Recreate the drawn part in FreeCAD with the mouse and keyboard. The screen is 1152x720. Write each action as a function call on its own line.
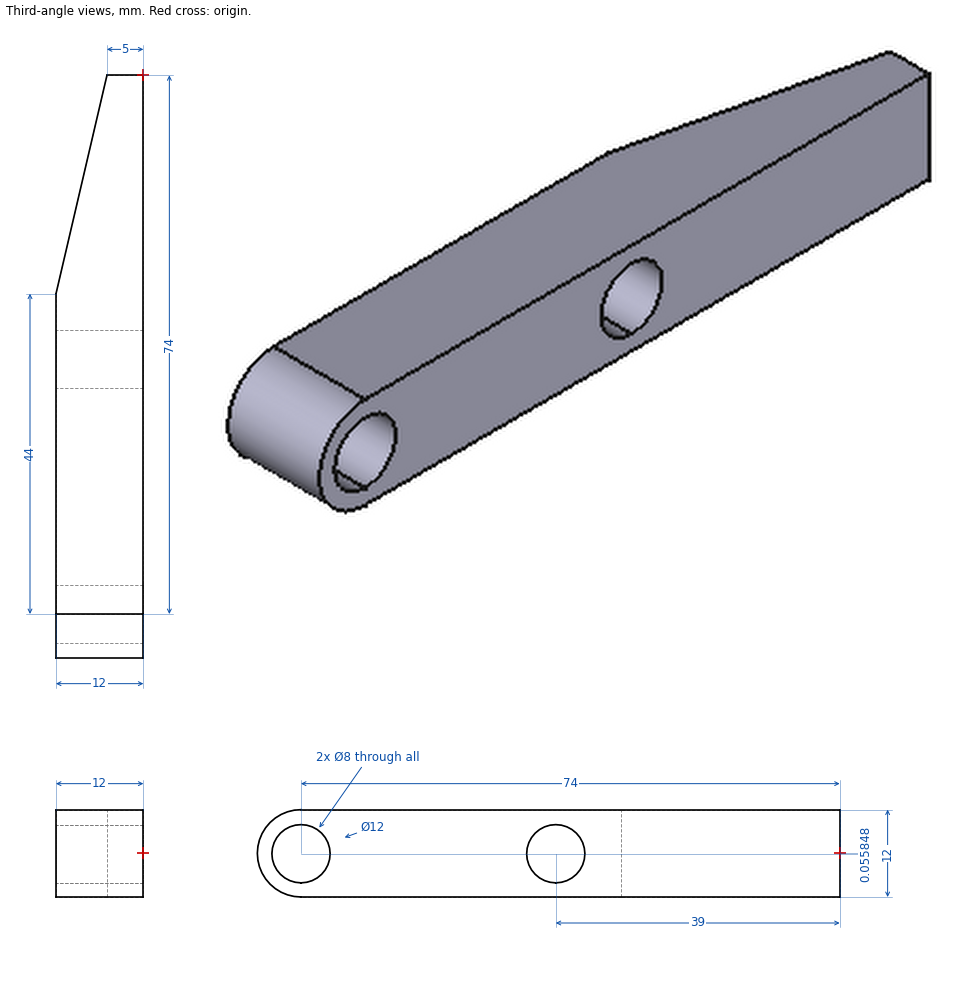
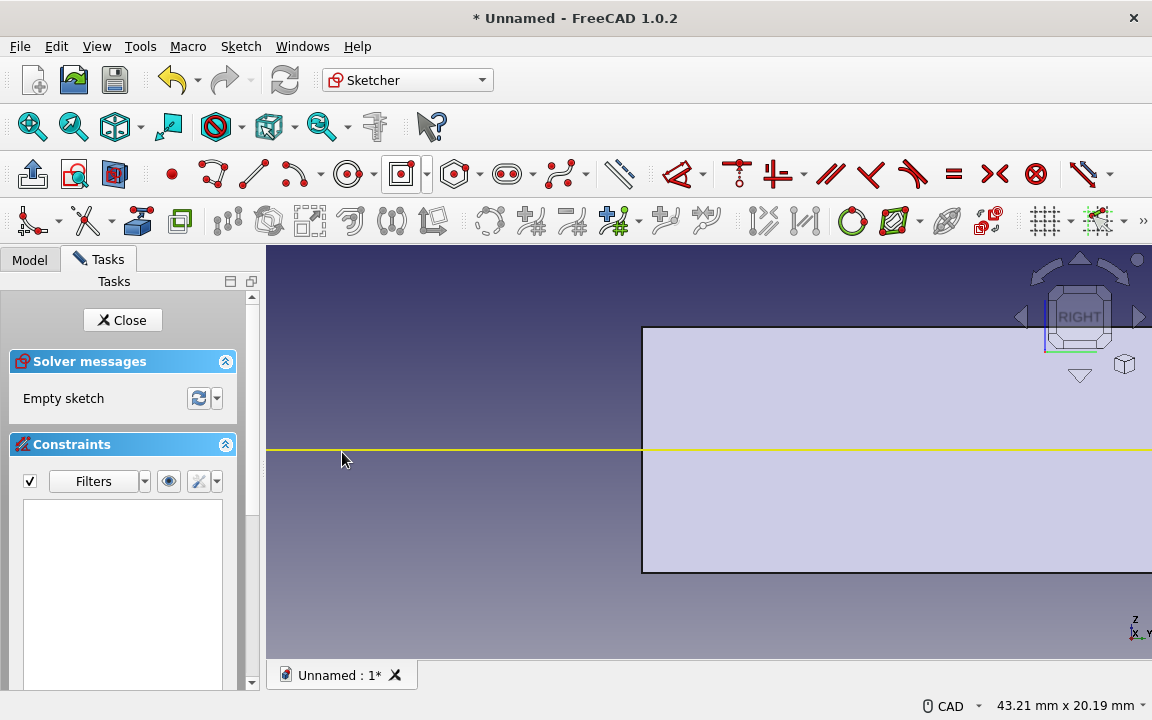
key(g)
key(c)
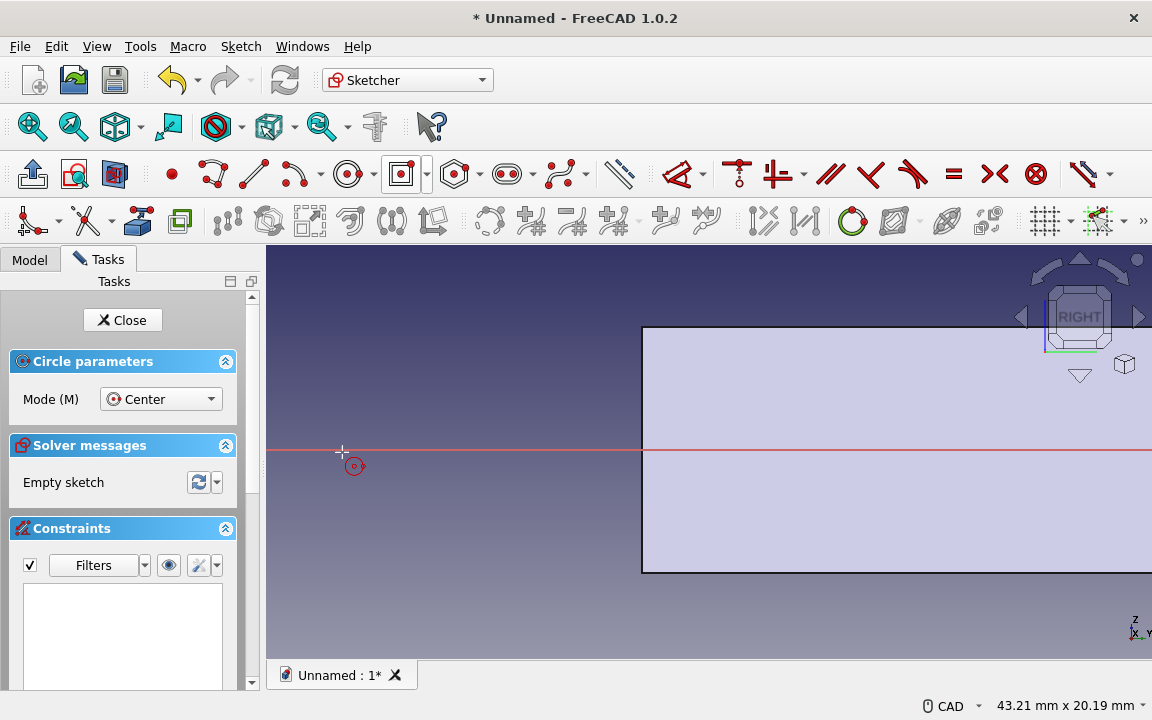
click(642, 450)
move(729, 363)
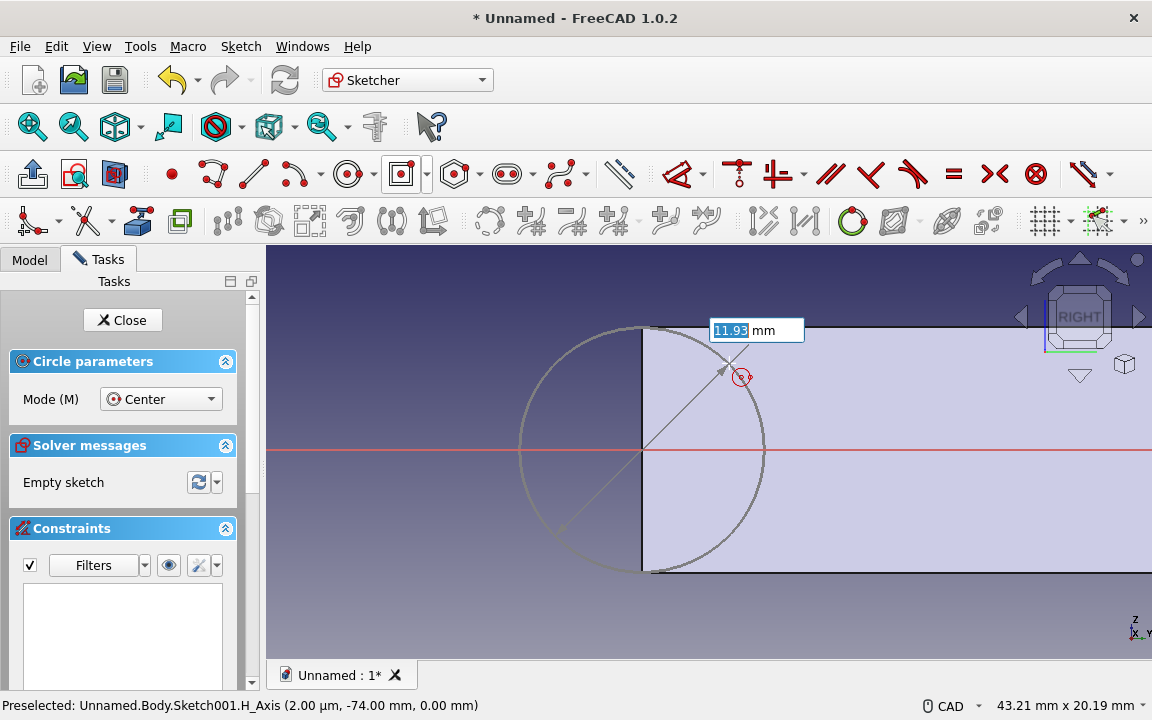
text(12)
key(Return)
key(Escape)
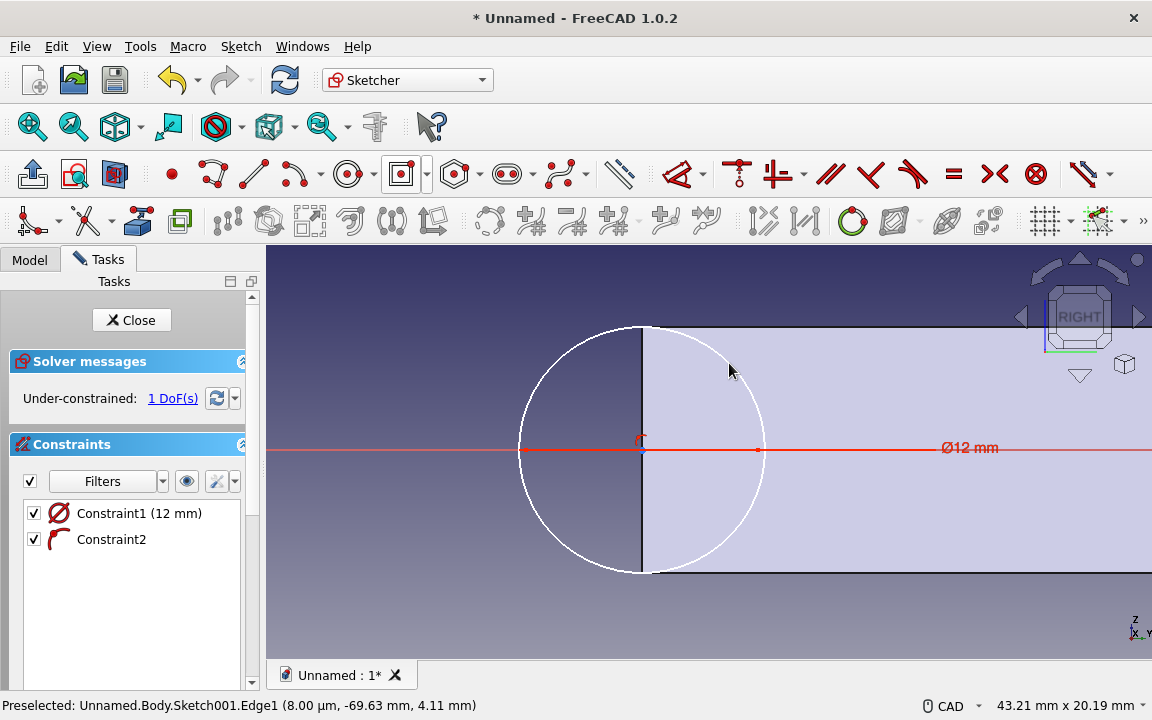
click(642, 450)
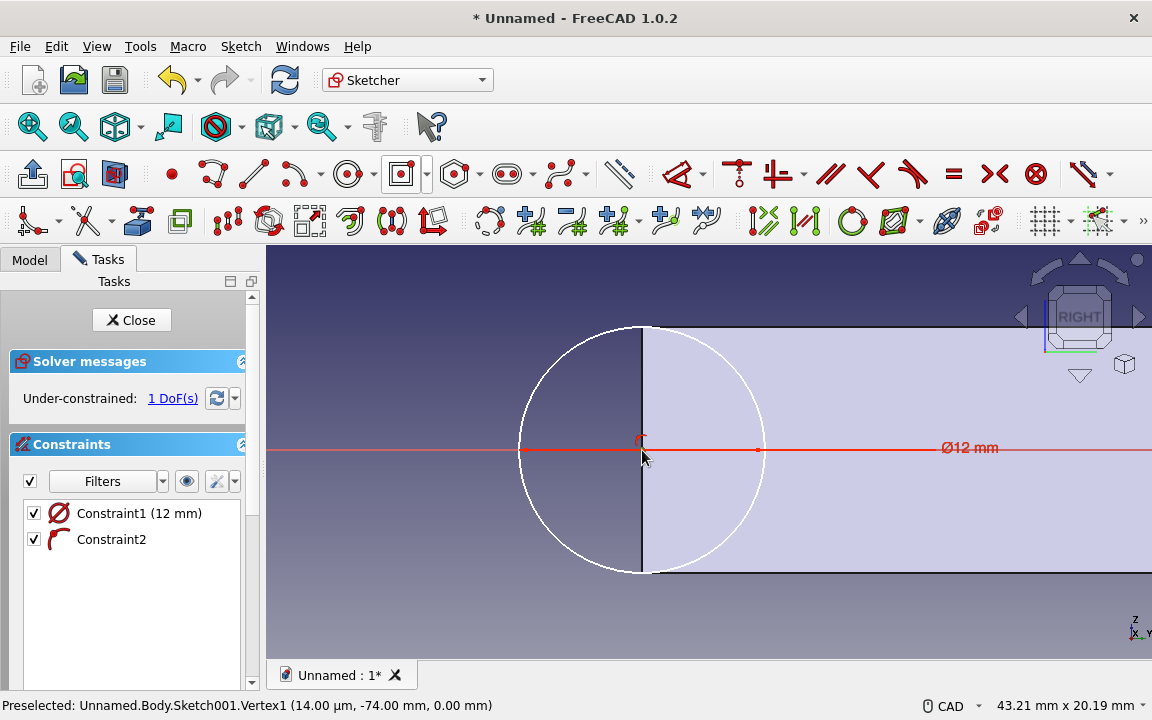
key(l)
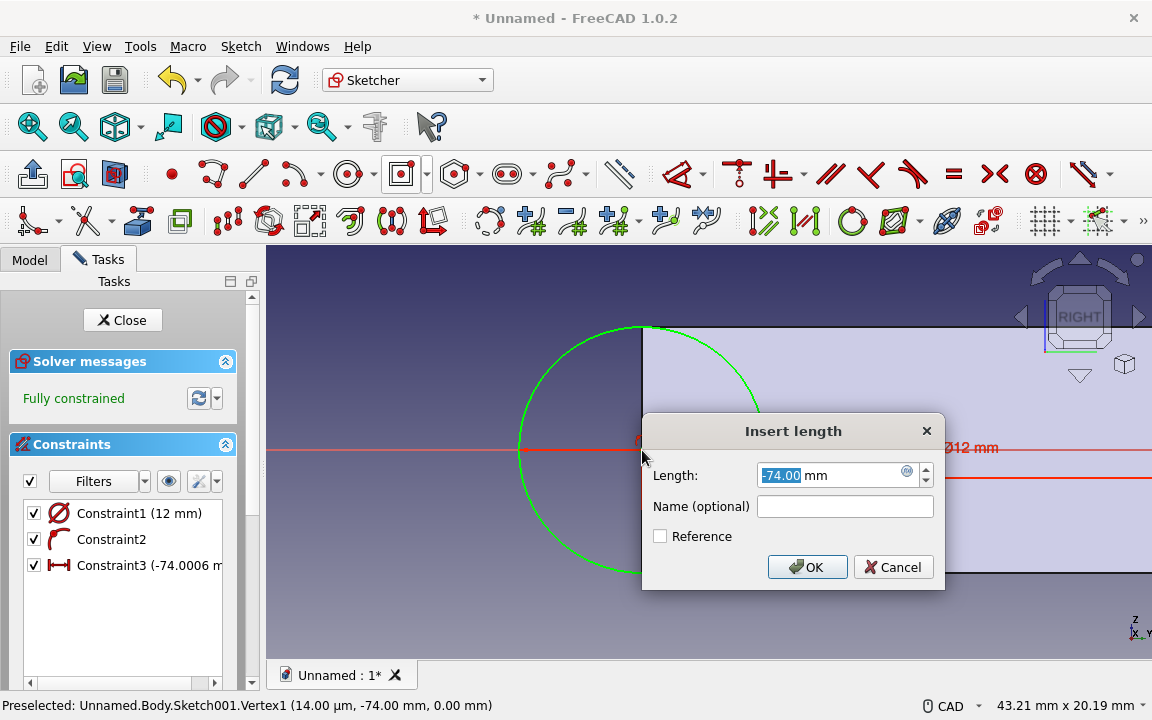
text(-74)
key(Return)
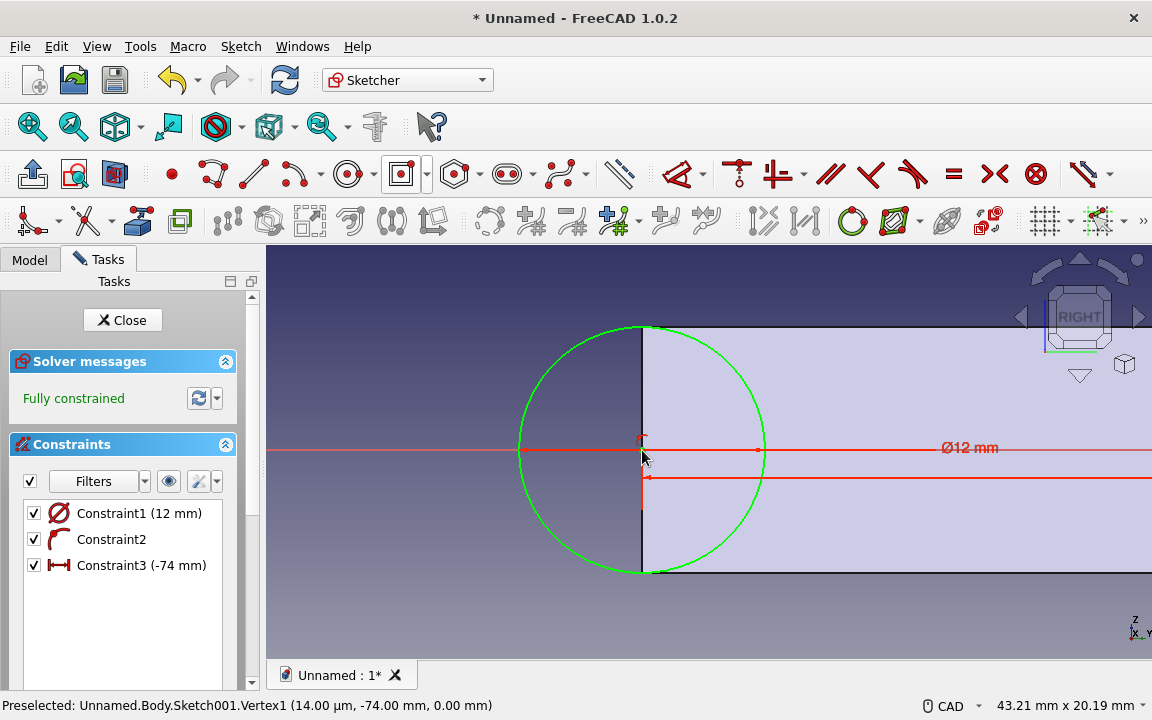
click(123, 320)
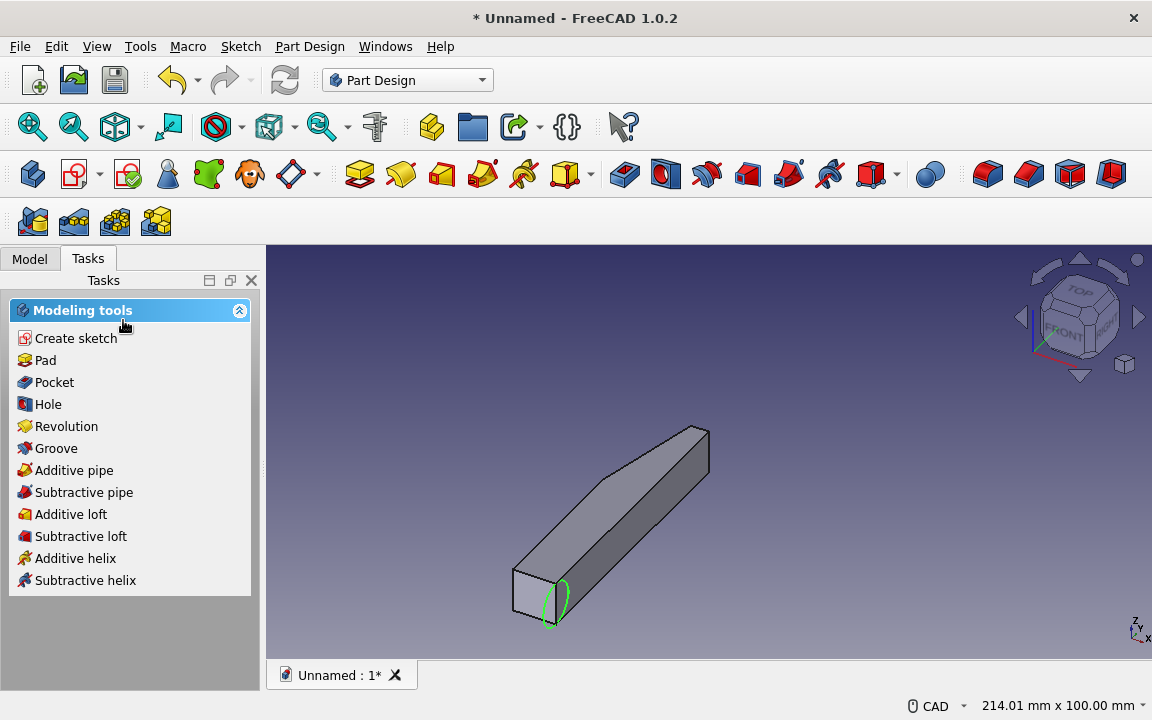
click(360, 174)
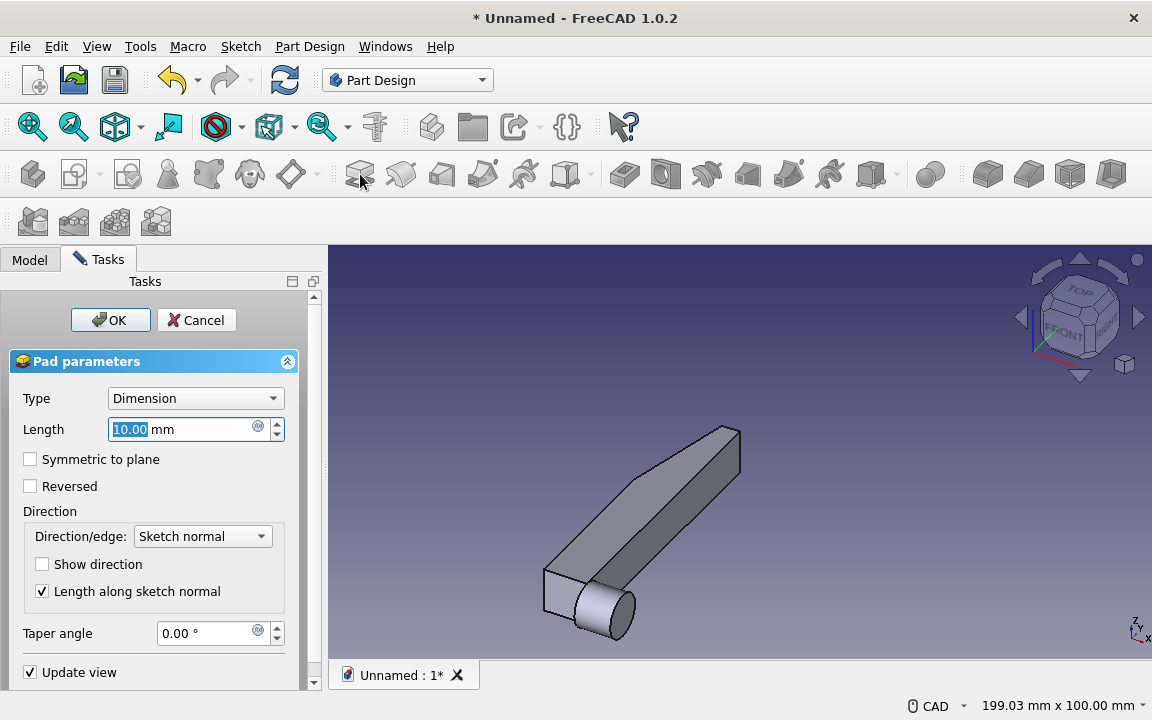
text(12)
key(Tab)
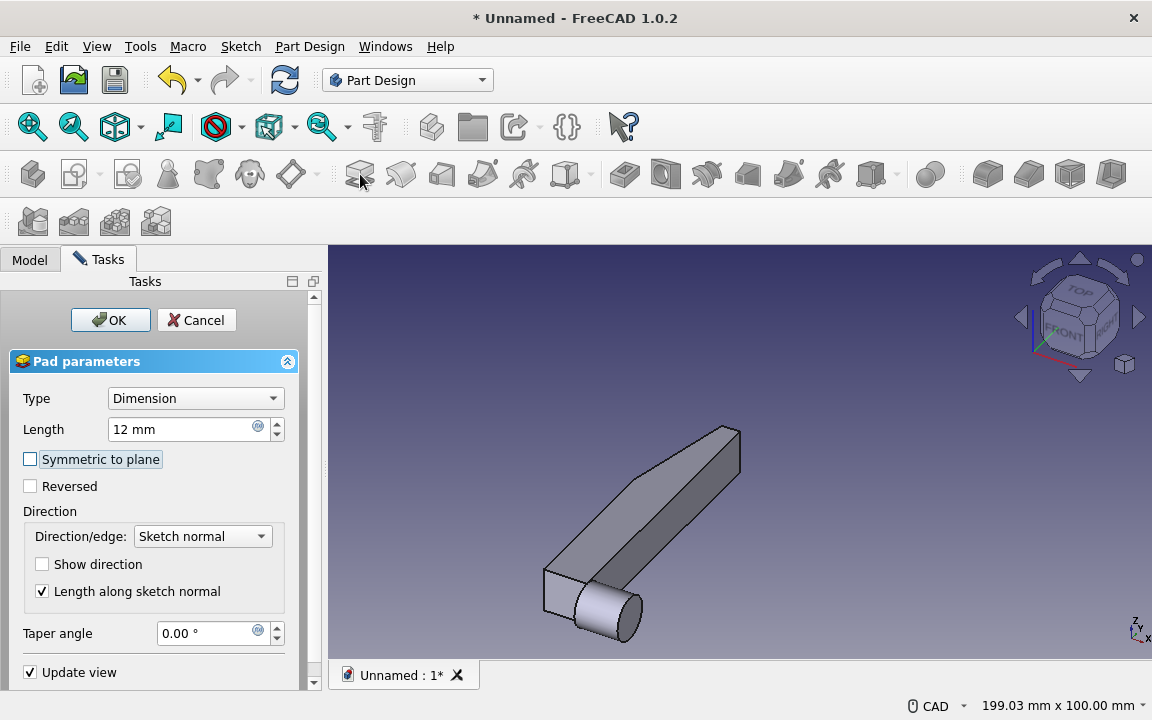
click(31, 486)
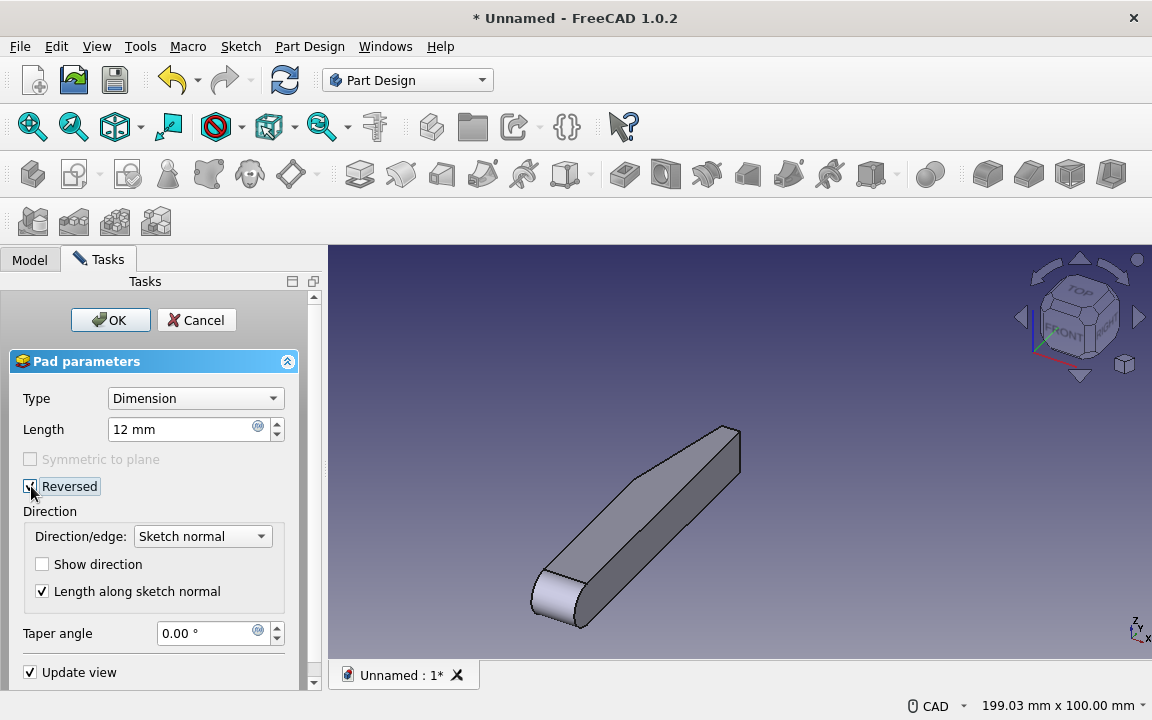
click(111, 320)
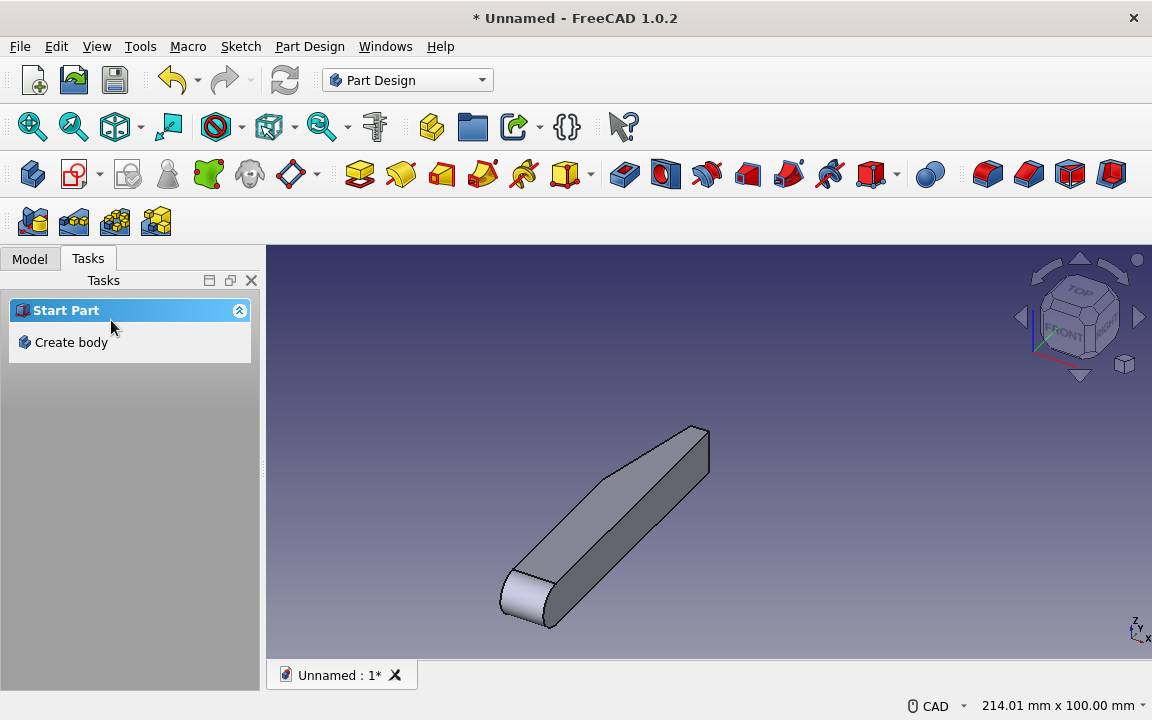
click(674, 486)